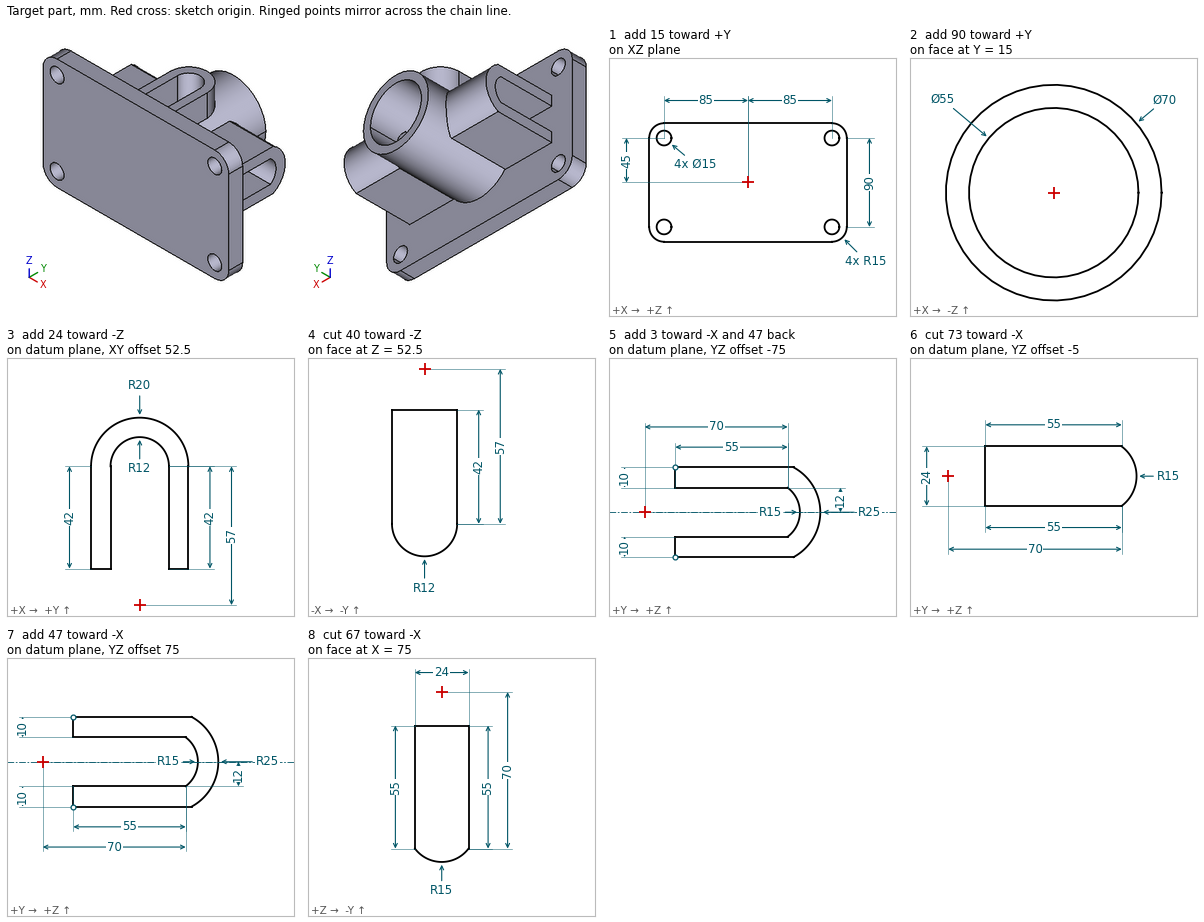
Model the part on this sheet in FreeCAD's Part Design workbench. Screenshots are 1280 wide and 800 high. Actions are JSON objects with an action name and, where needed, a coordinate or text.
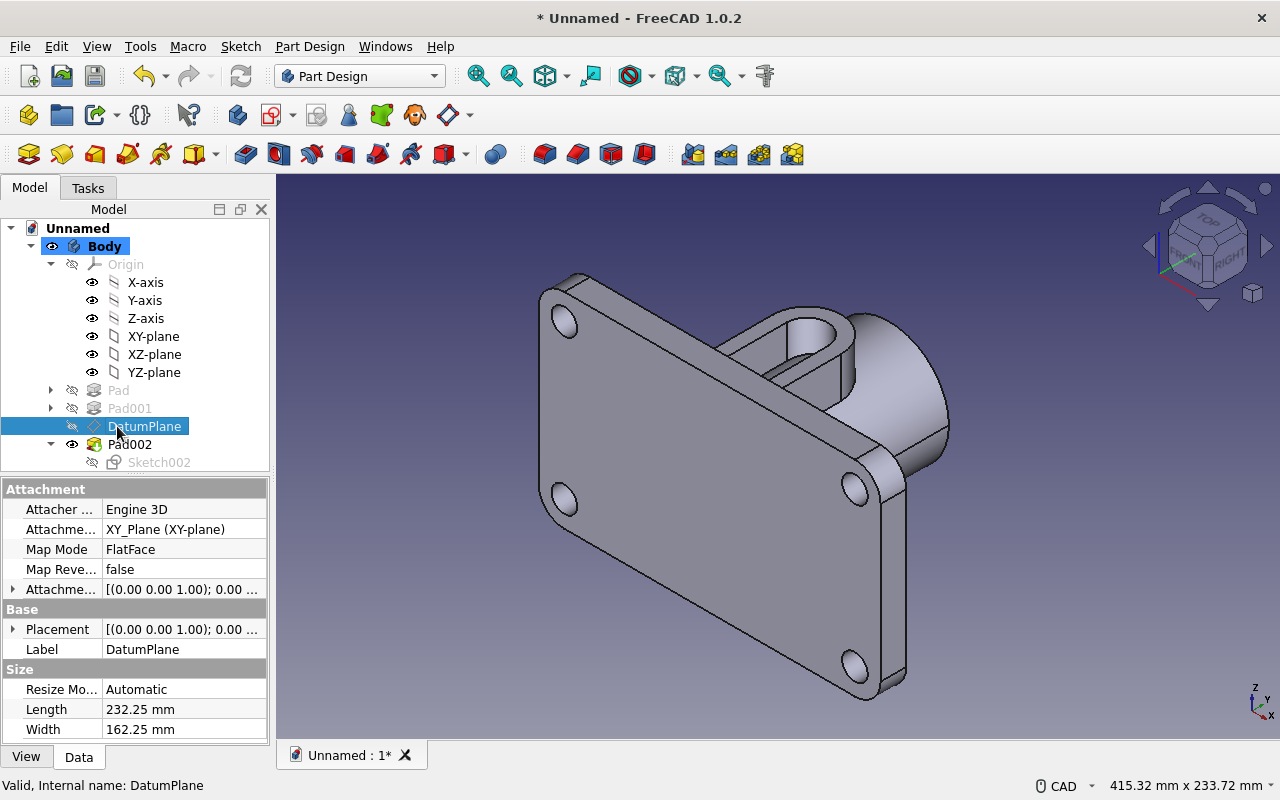
{"action": "left_click", "coordinate": [479, 76]}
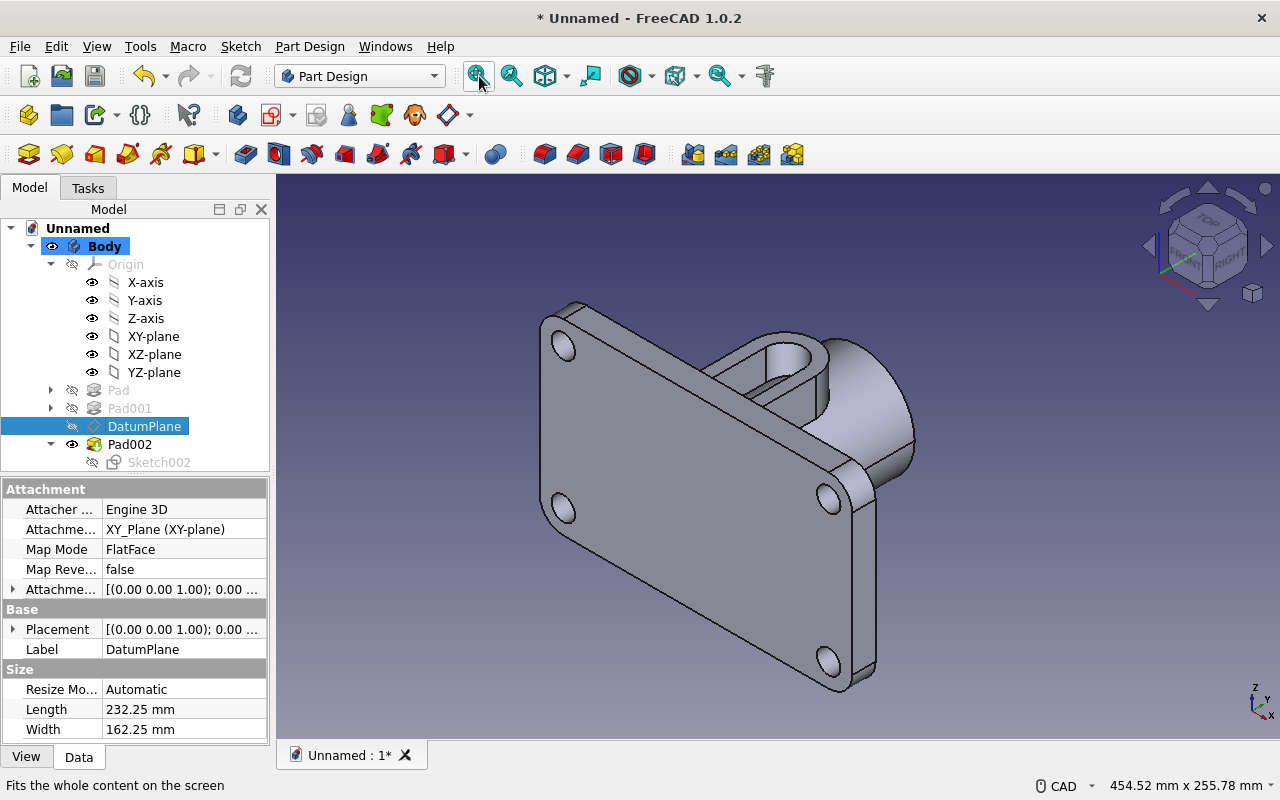
{"action": "key", "text": "2"}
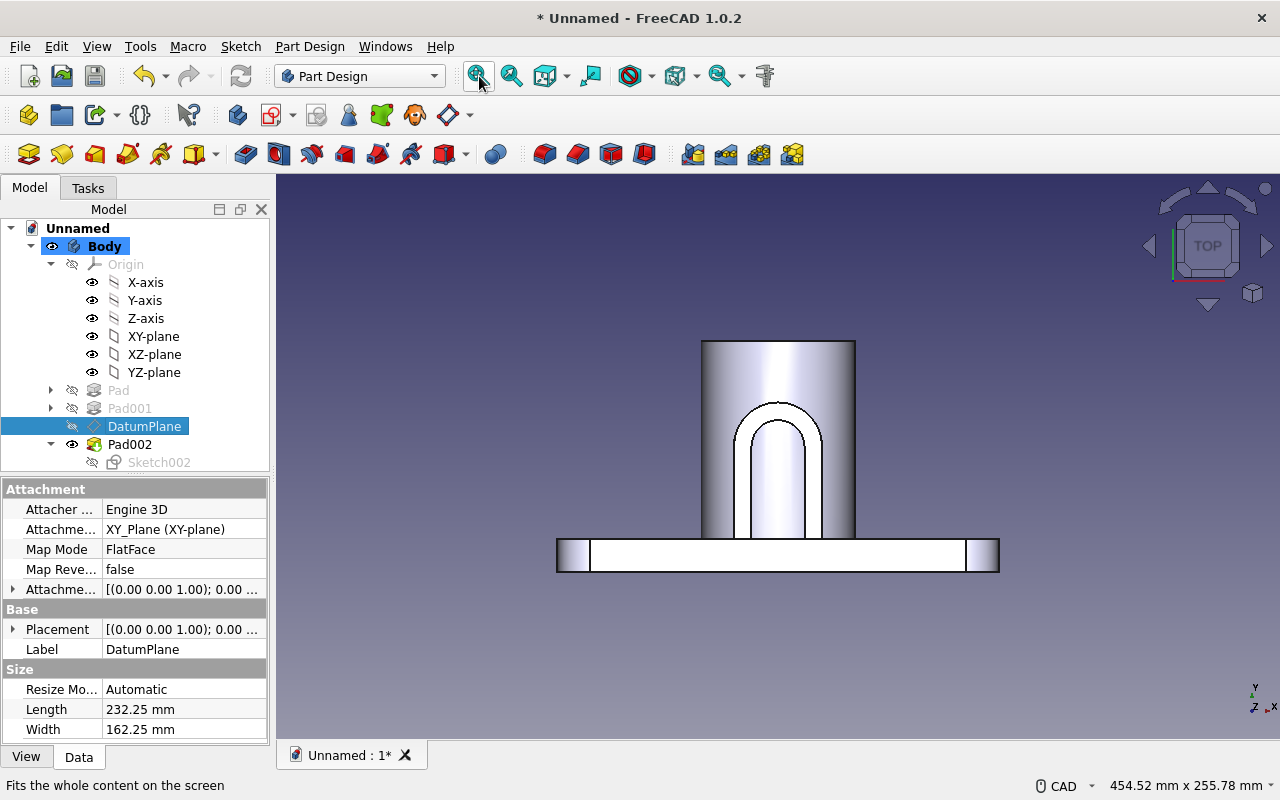
{"action": "key", "text": "v f"}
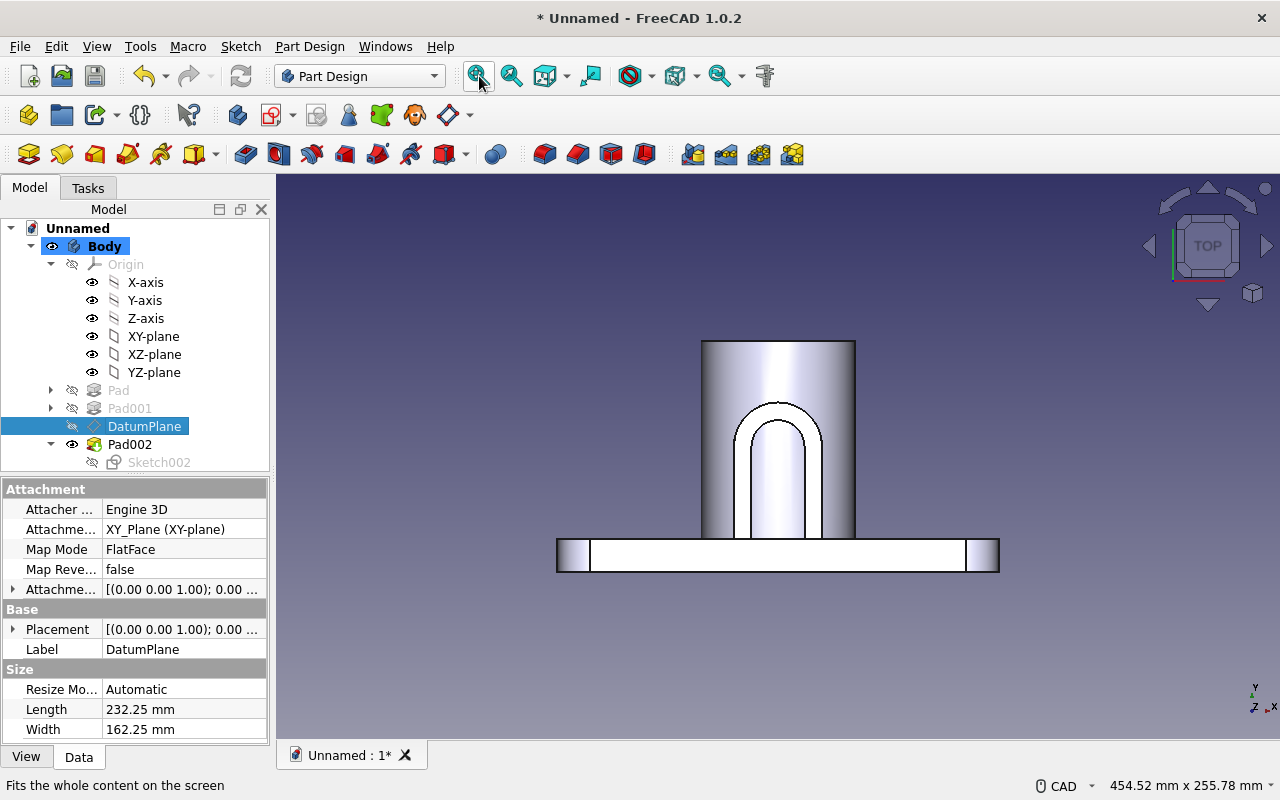
{"action": "left_click", "coordinate": [778, 411]}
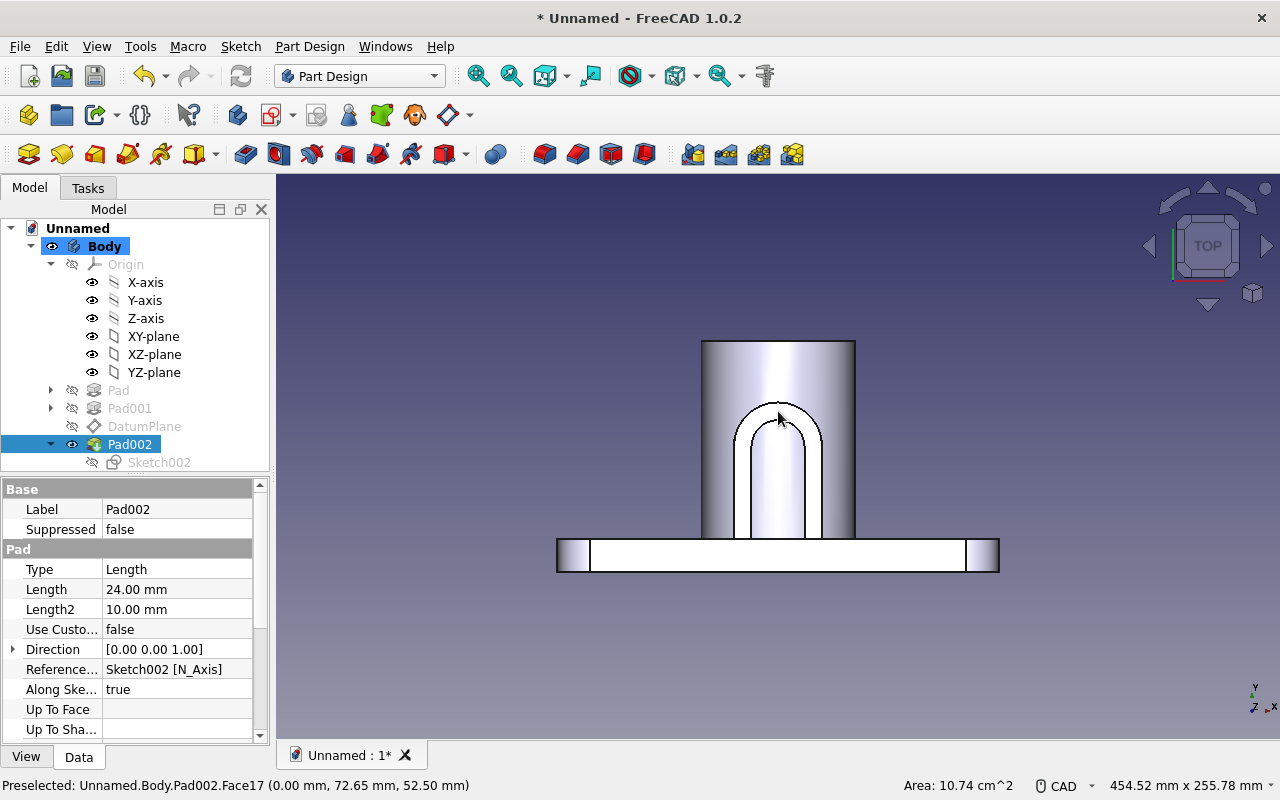
{"action": "left_click", "coordinate": [270, 116]}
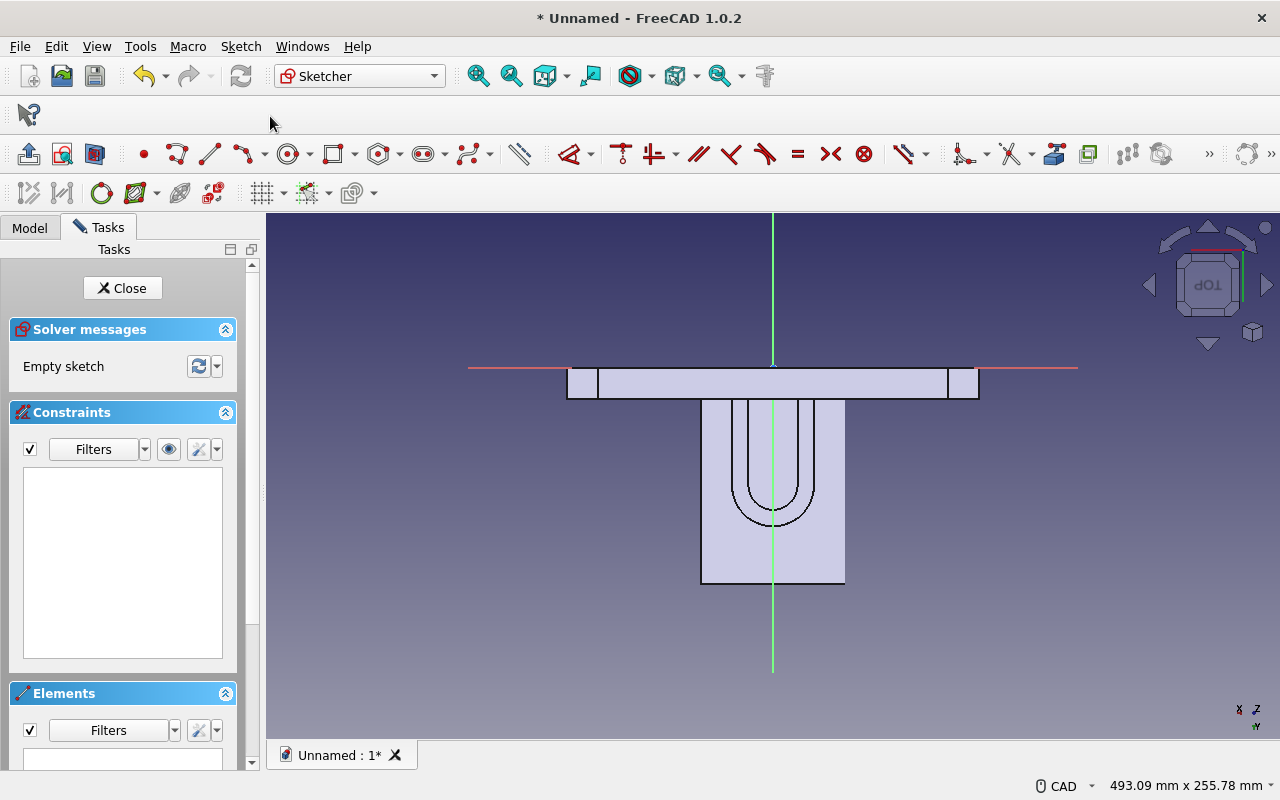
{"action": "scroll", "coordinate": [829, 409], "scroll_direction": "up", "scroll_amount": 4}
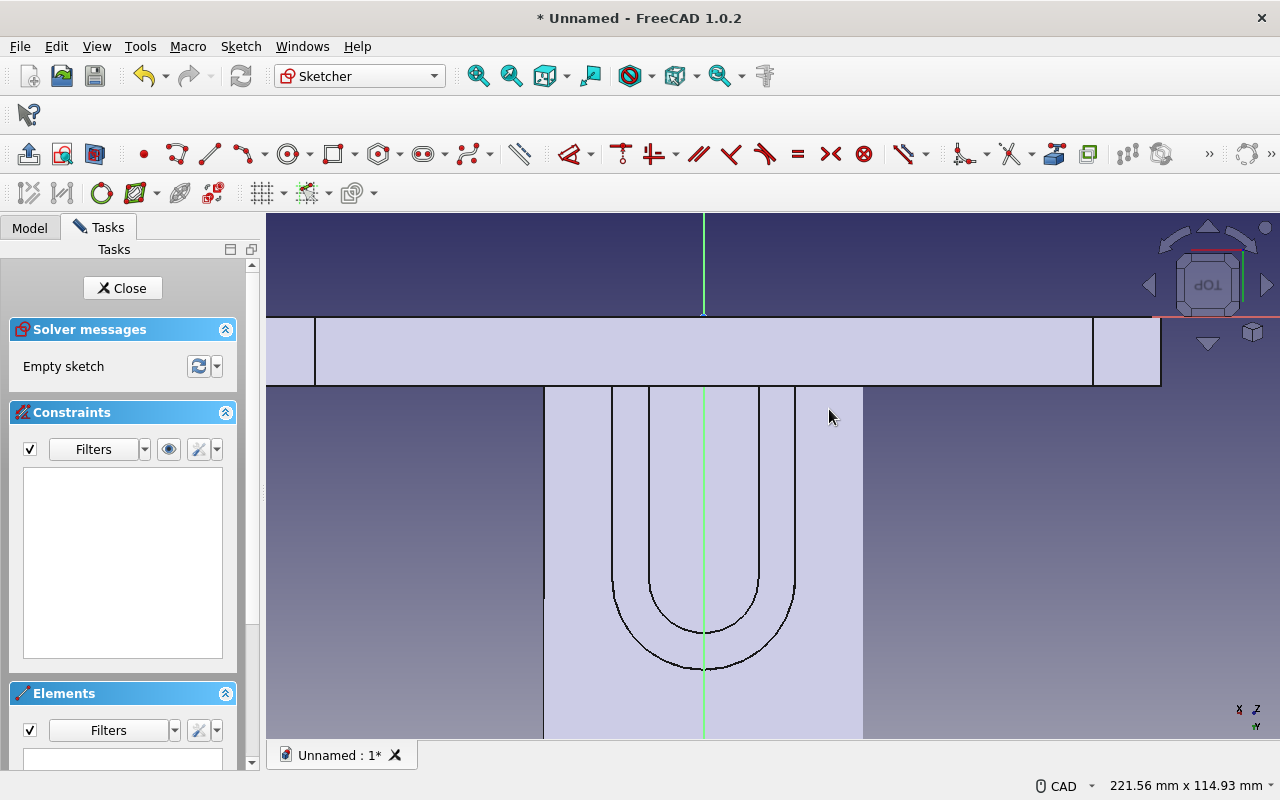
{"action": "key", "text": "g m"}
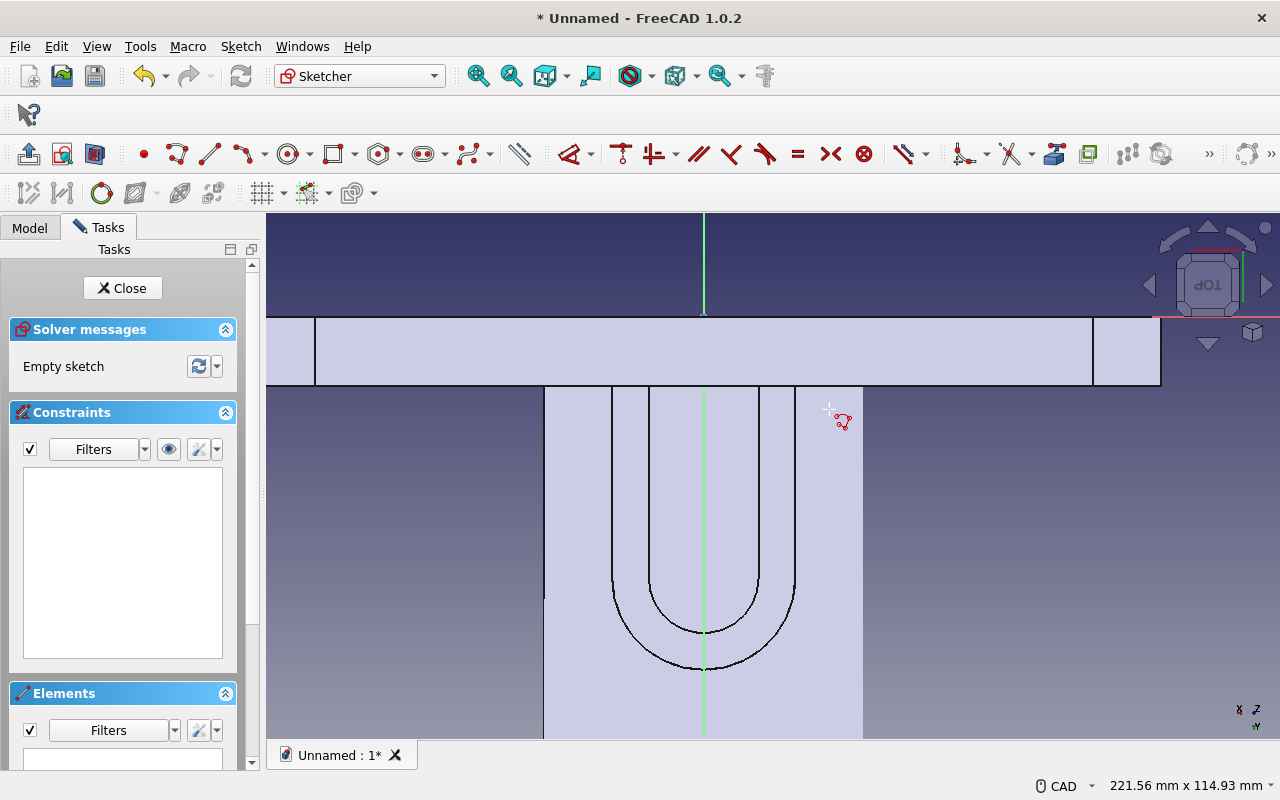
{"action": "left_click", "coordinate": [759, 578]}
{"action": "left_click", "coordinate": [759, 386]}
{"action": "left_click", "coordinate": [649, 386]}
{"action": "left_click", "coordinate": [649, 578]}
{"action": "right_click", "coordinate": [649, 578]}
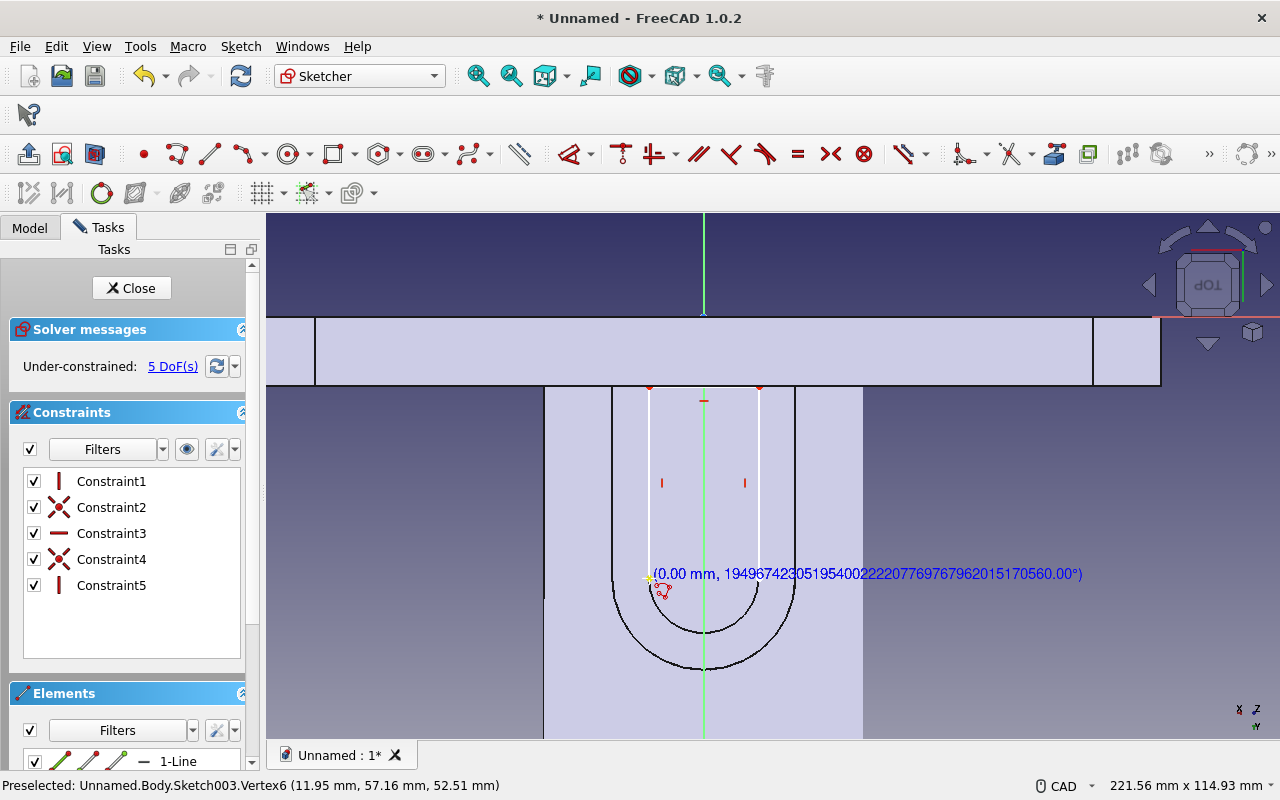
{"action": "left_click", "coordinate": [242, 154]}